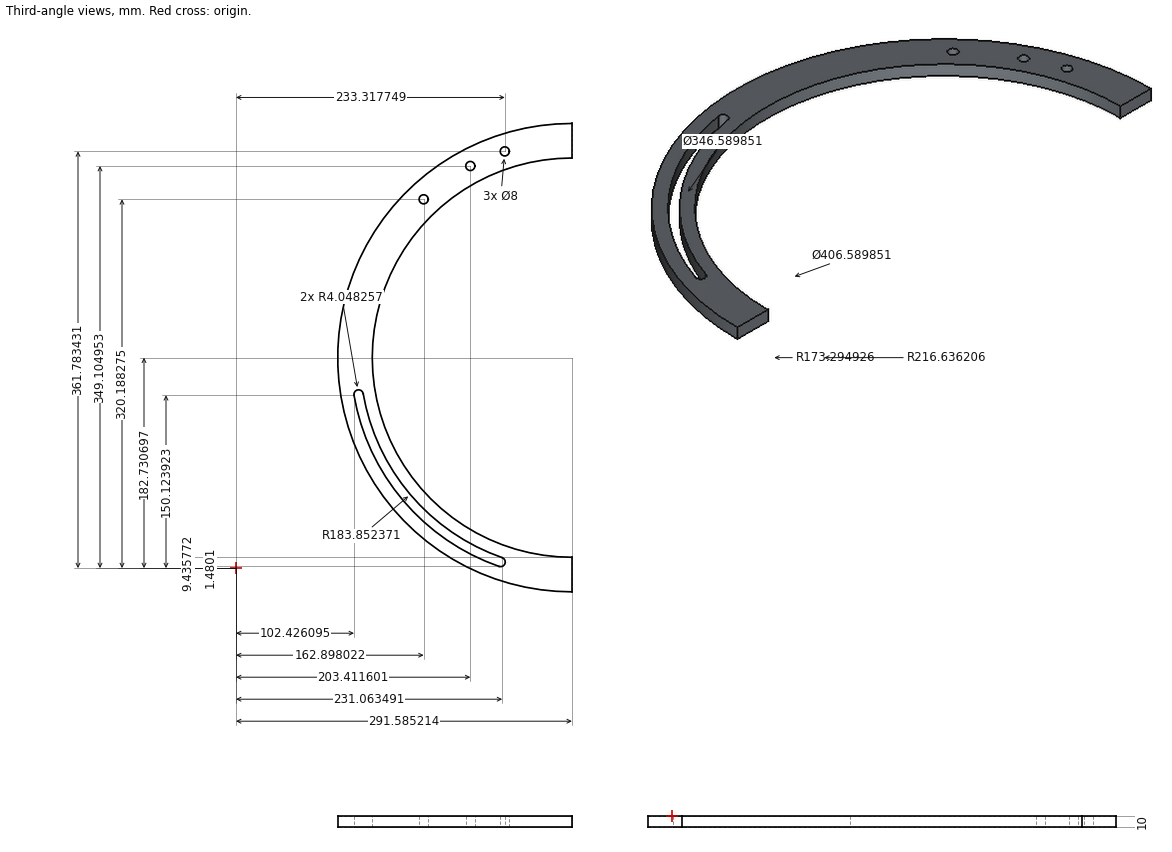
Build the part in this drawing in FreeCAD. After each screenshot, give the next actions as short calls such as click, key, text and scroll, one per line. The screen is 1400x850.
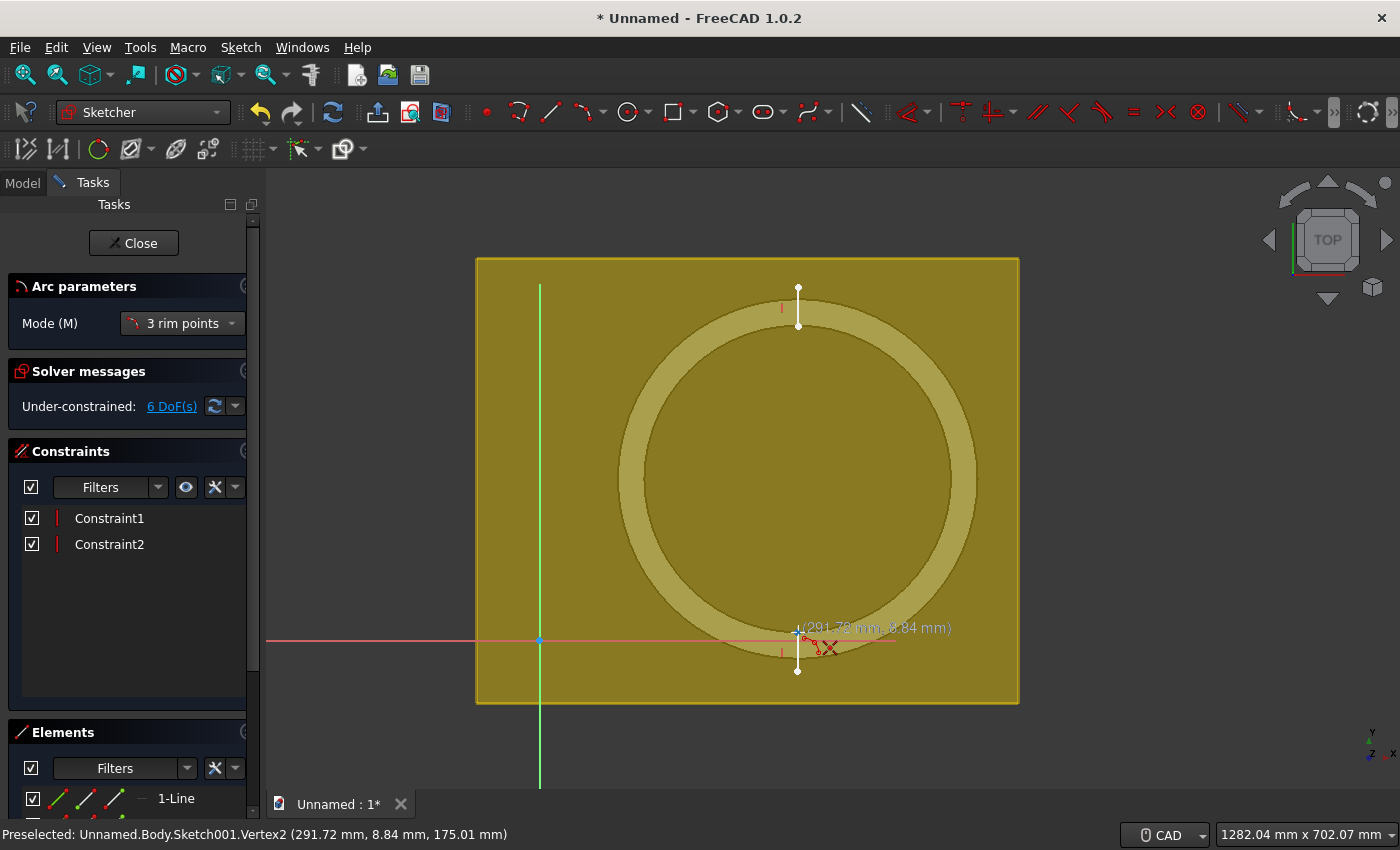
click(798, 327)
click(951, 479)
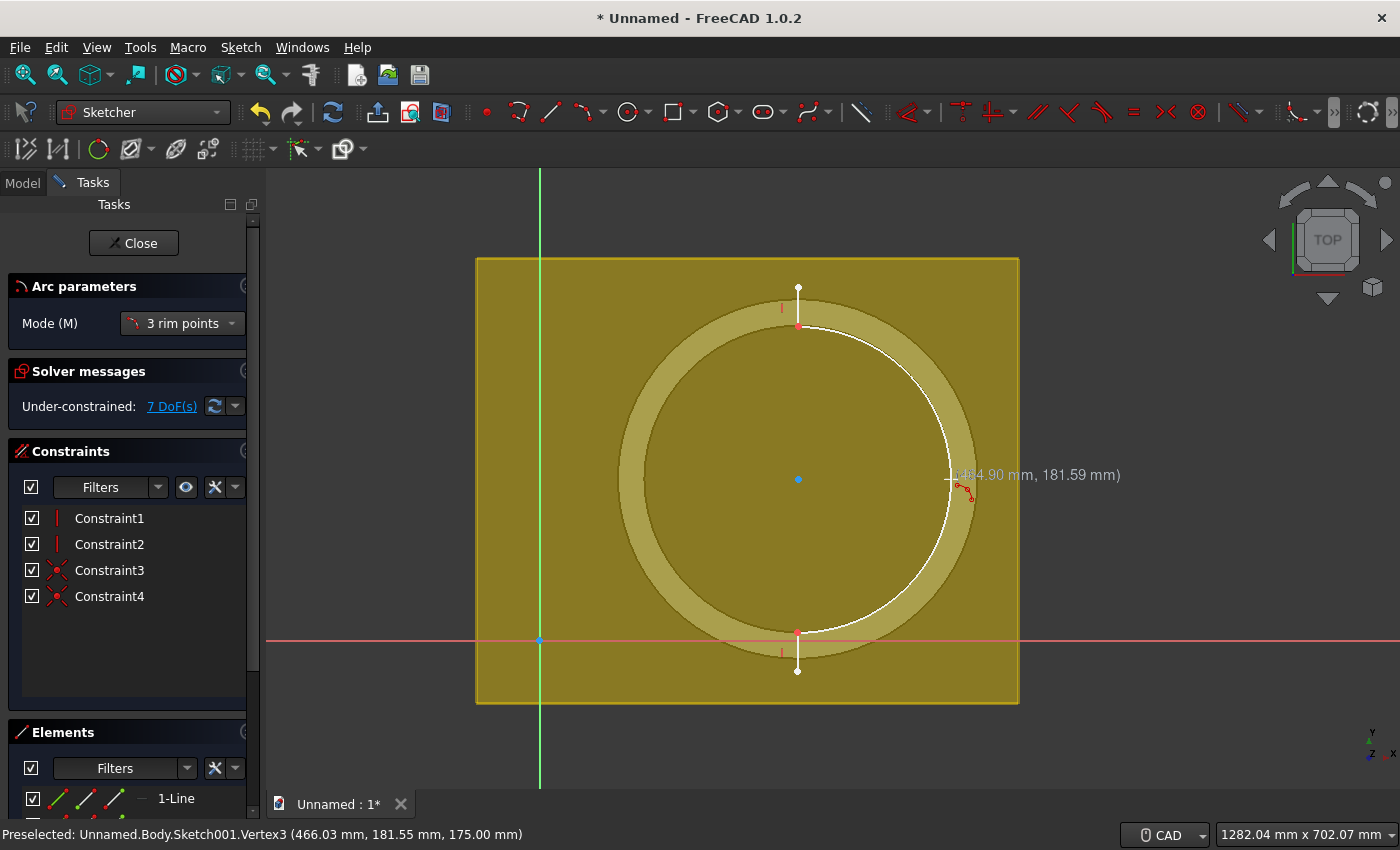
click(798, 288)
click(798, 672)
click(989, 479)
key(Escape)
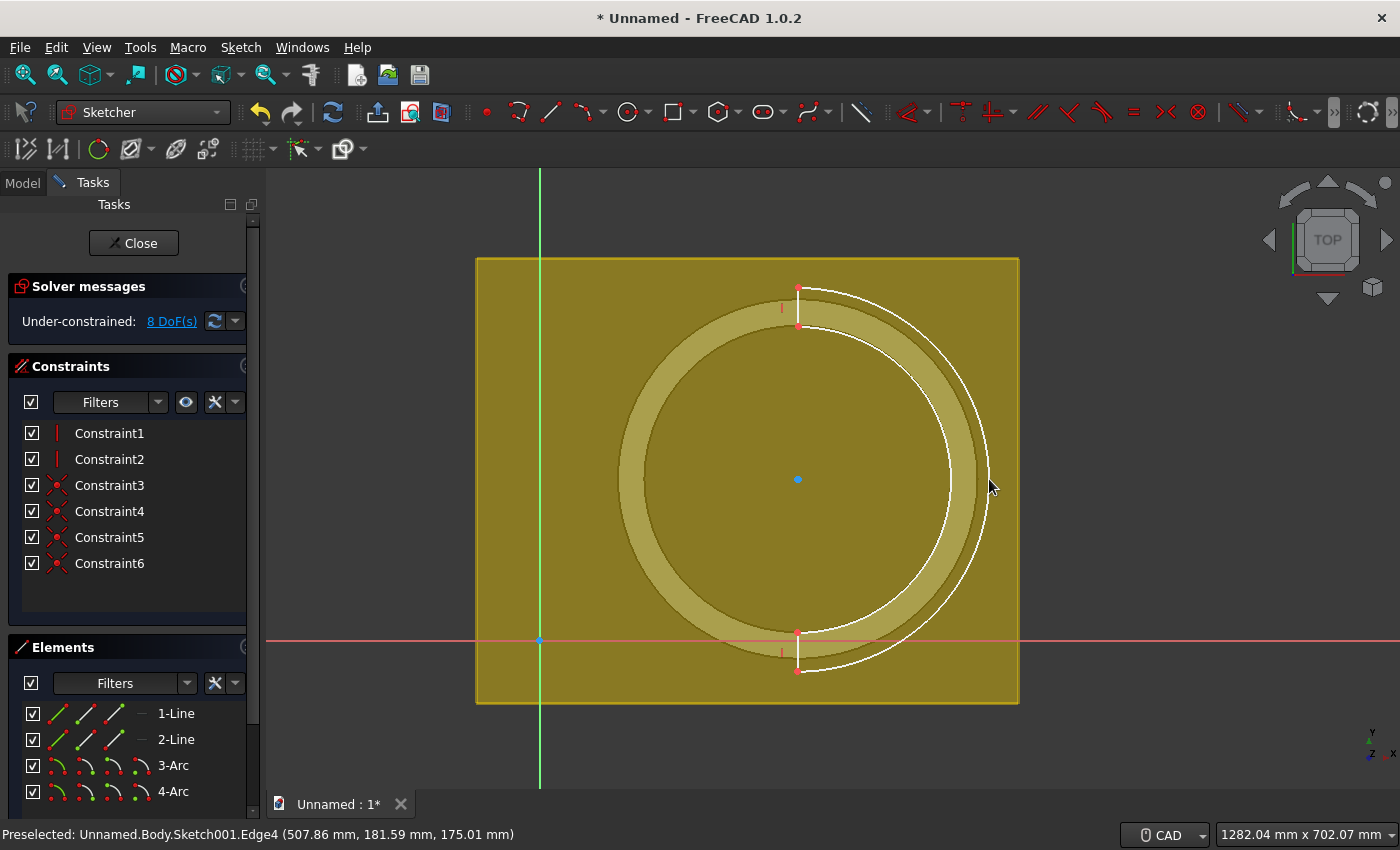
click(922, 570)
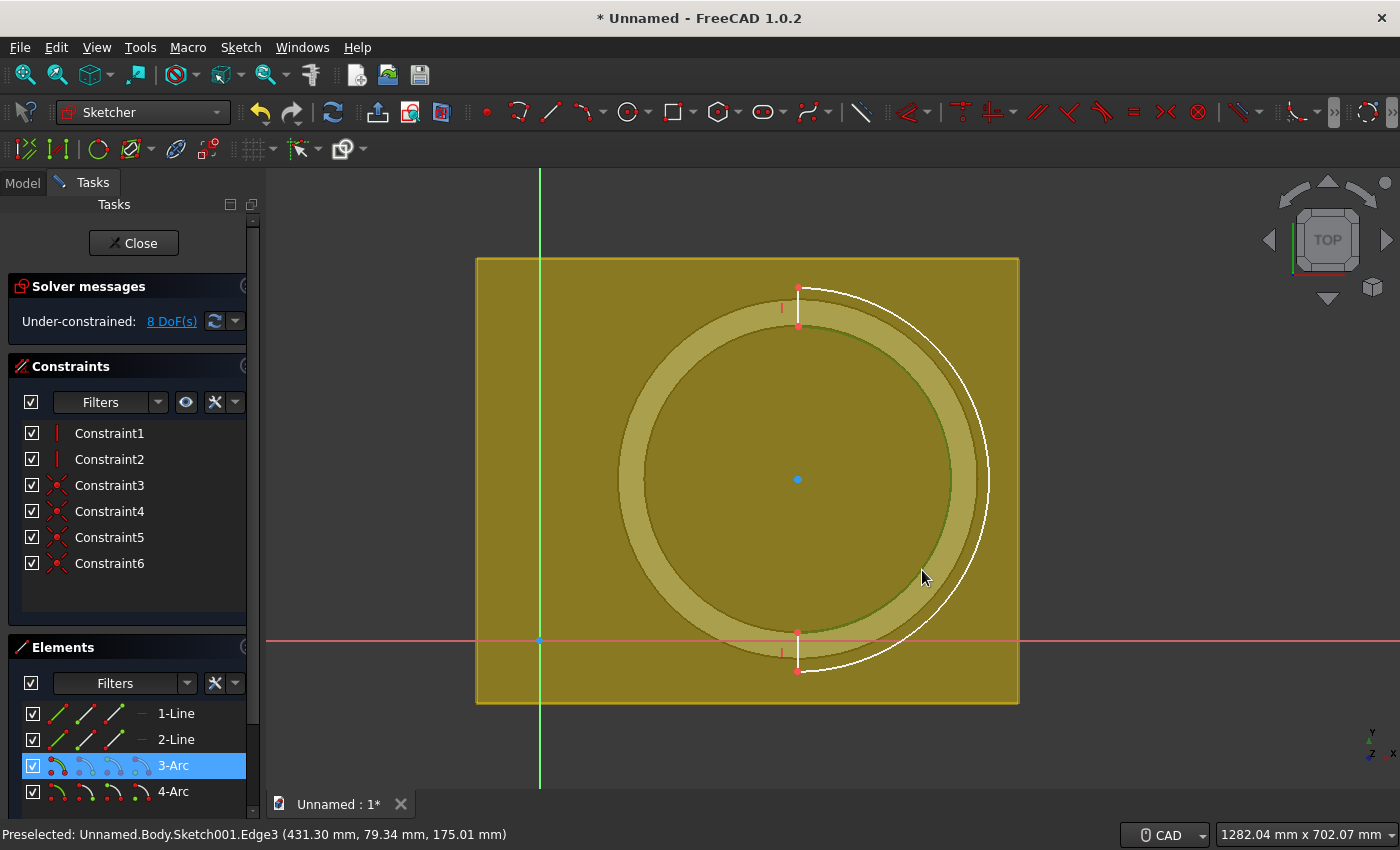
click(952, 593)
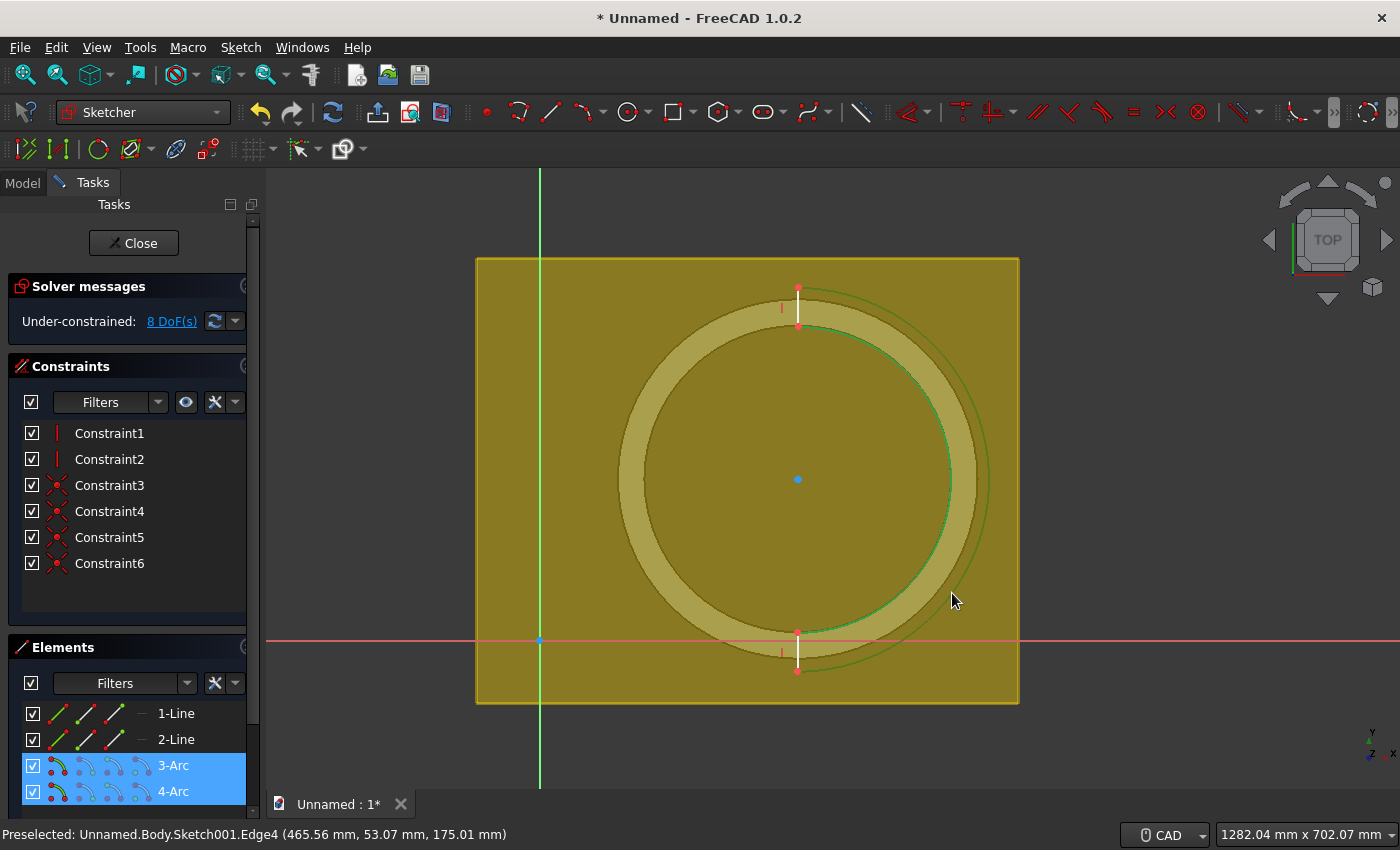
click(962, 112)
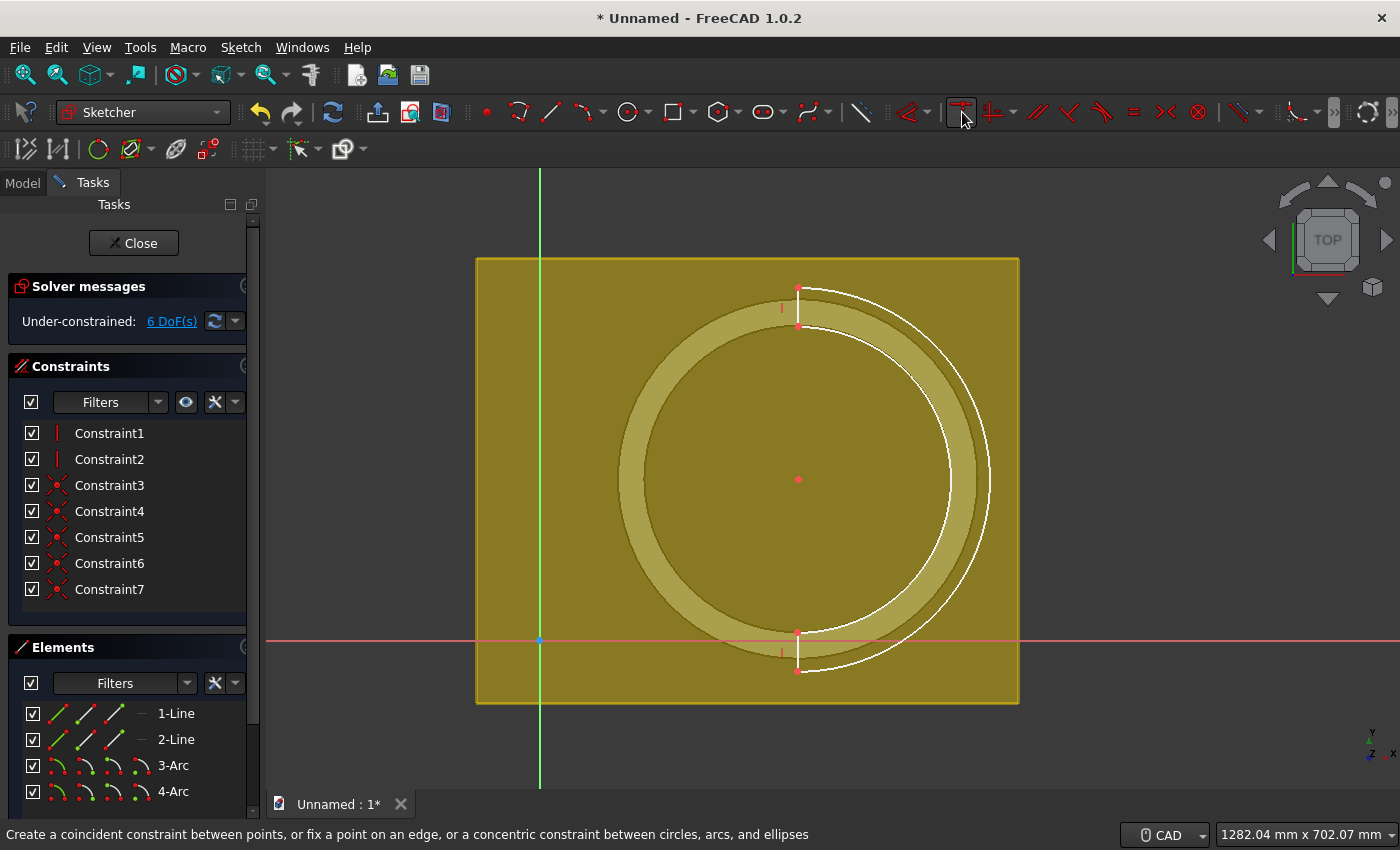
click(908, 112)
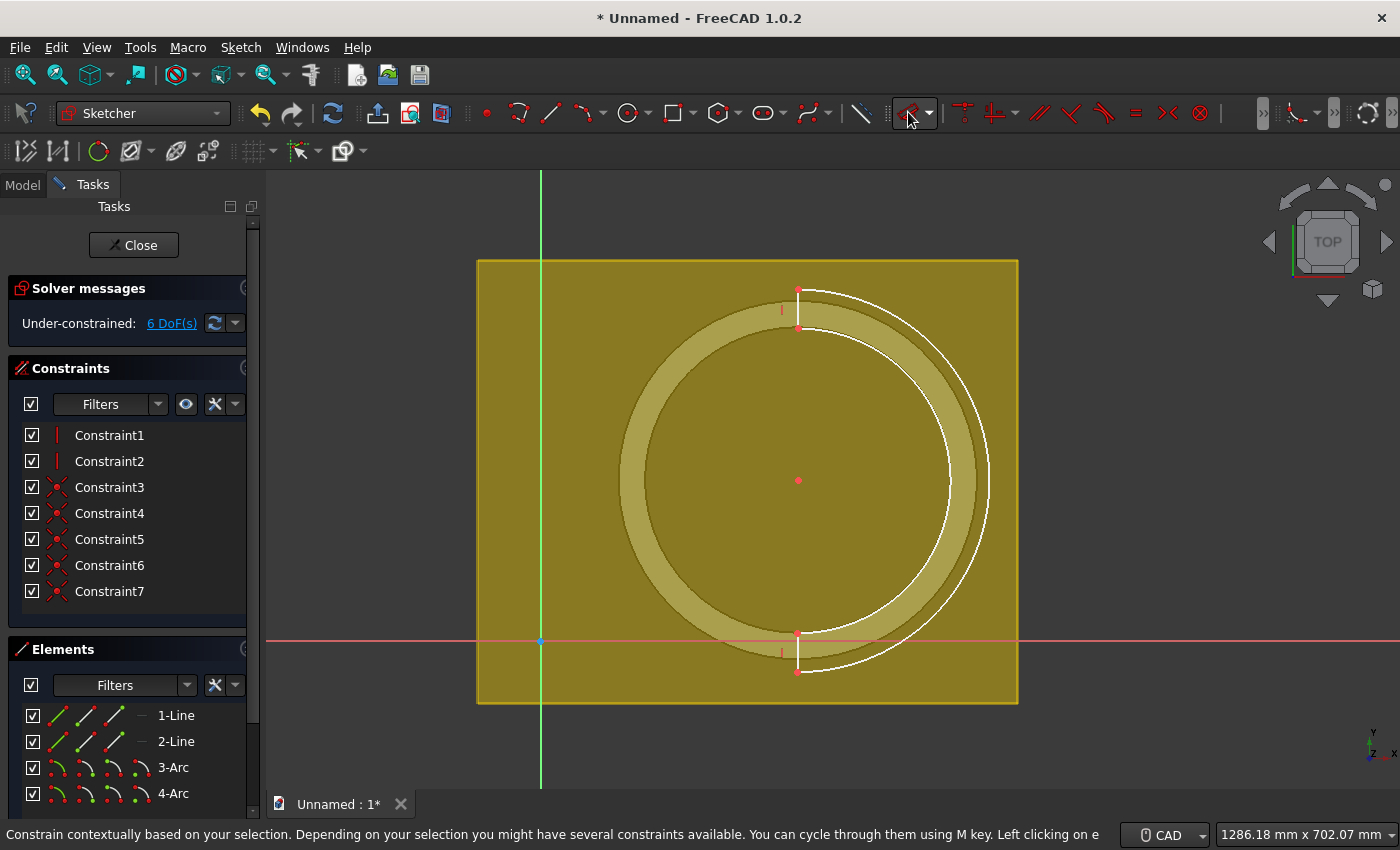
click(921, 571)
click(649, 372)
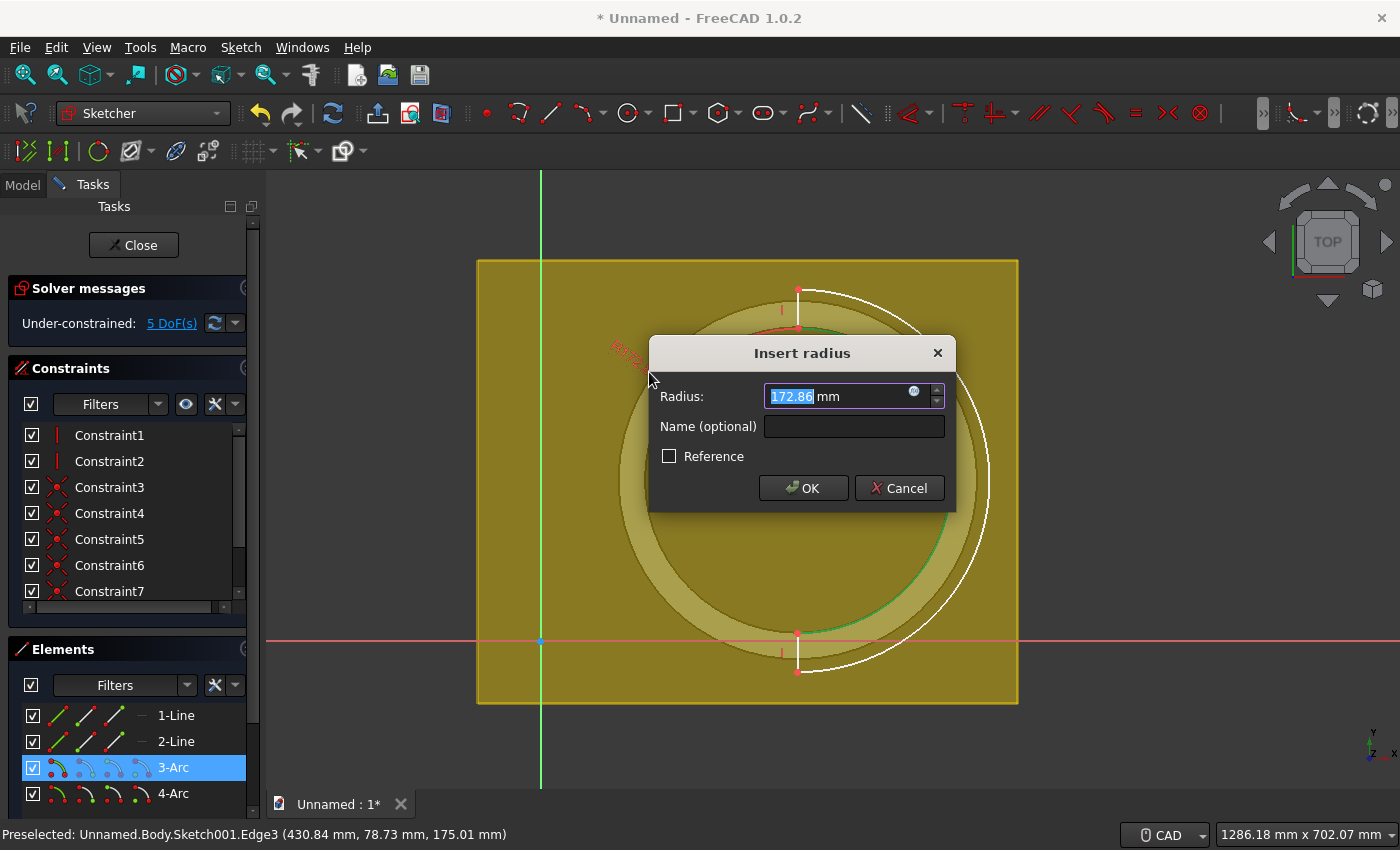
text(173.294926)
key(Return)